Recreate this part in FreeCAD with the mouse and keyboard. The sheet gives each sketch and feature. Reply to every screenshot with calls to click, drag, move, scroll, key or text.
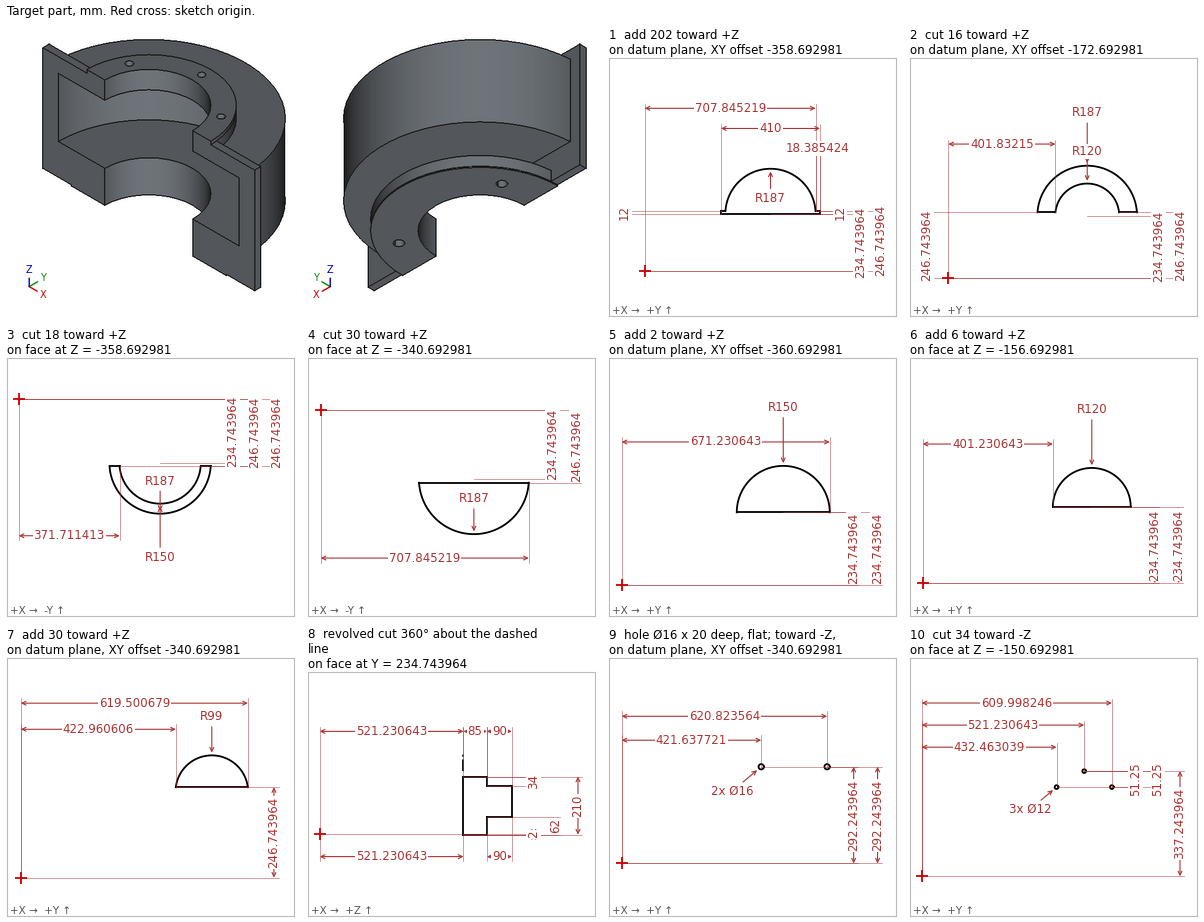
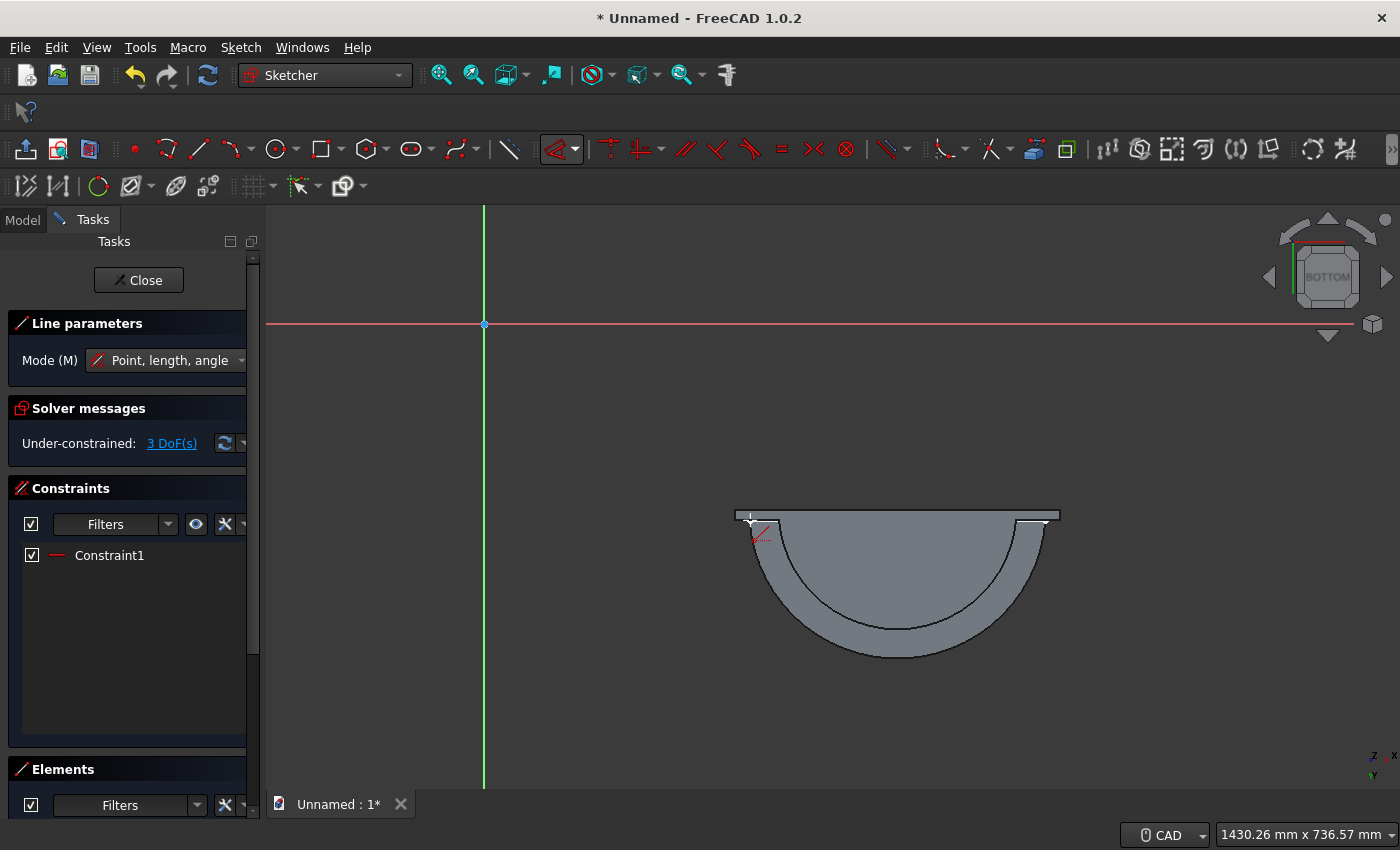
key(g)
key(3)
key(a)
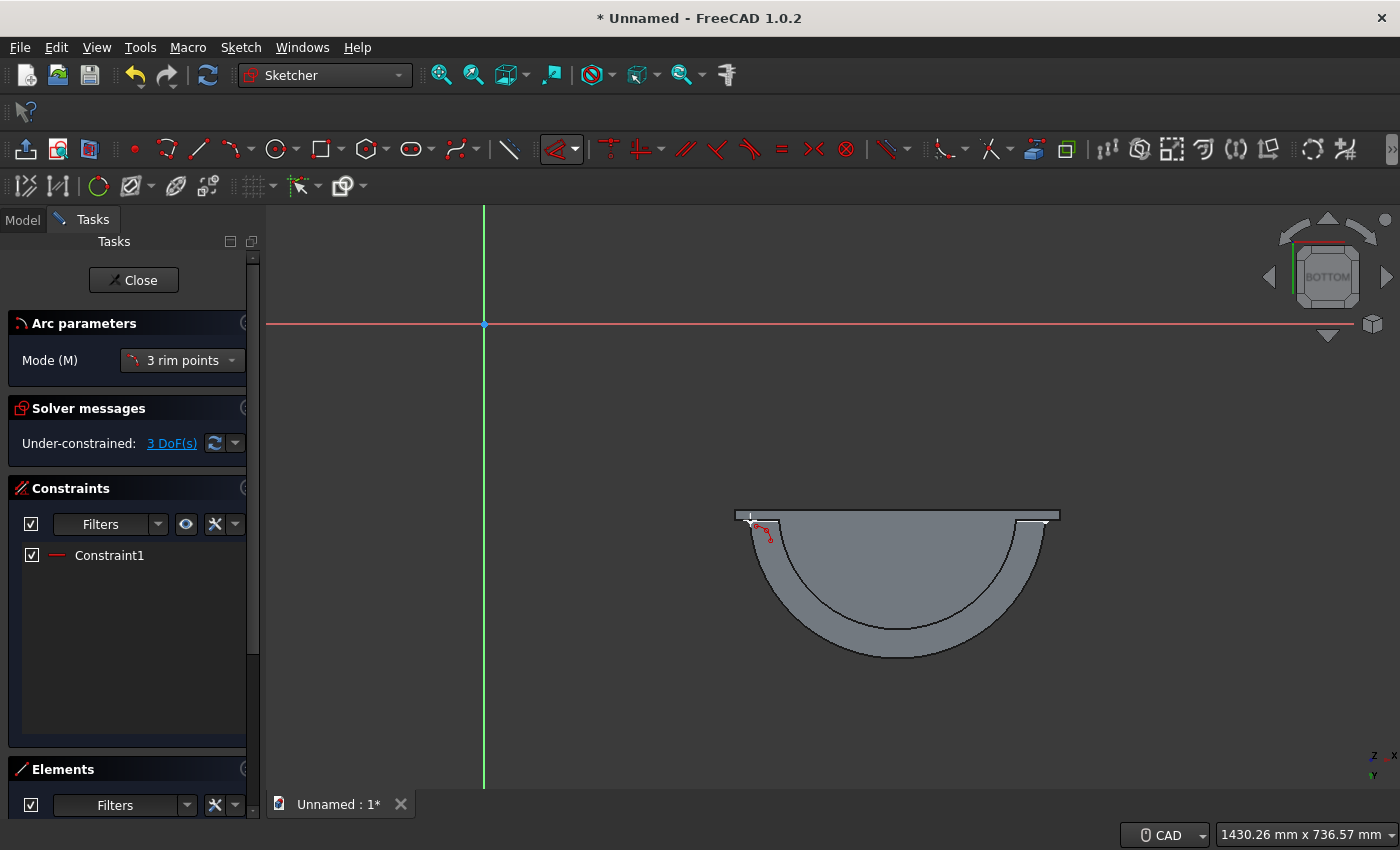
click(750, 521)
click(1045, 521)
click(898, 659)
key(Escape)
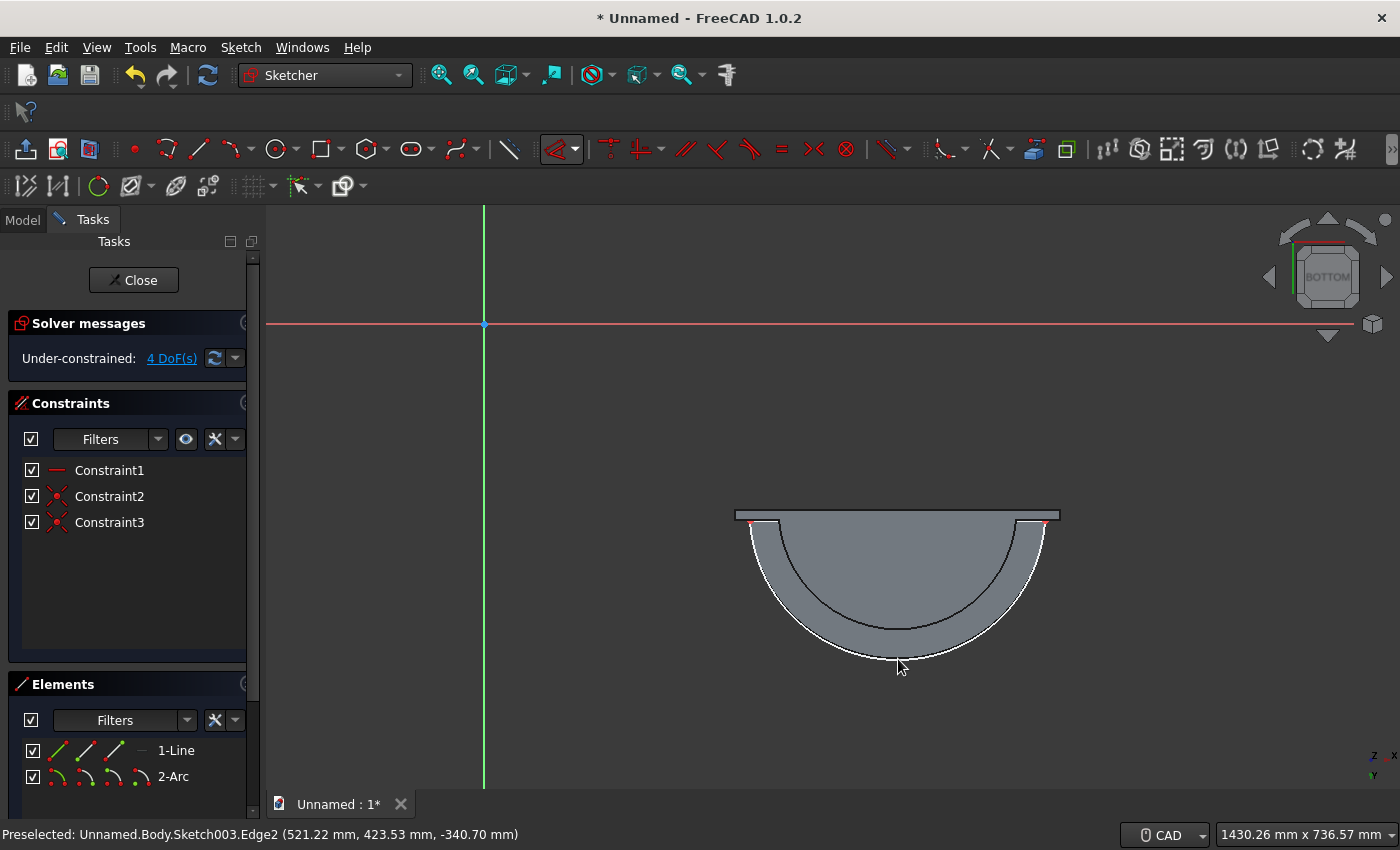
key(d)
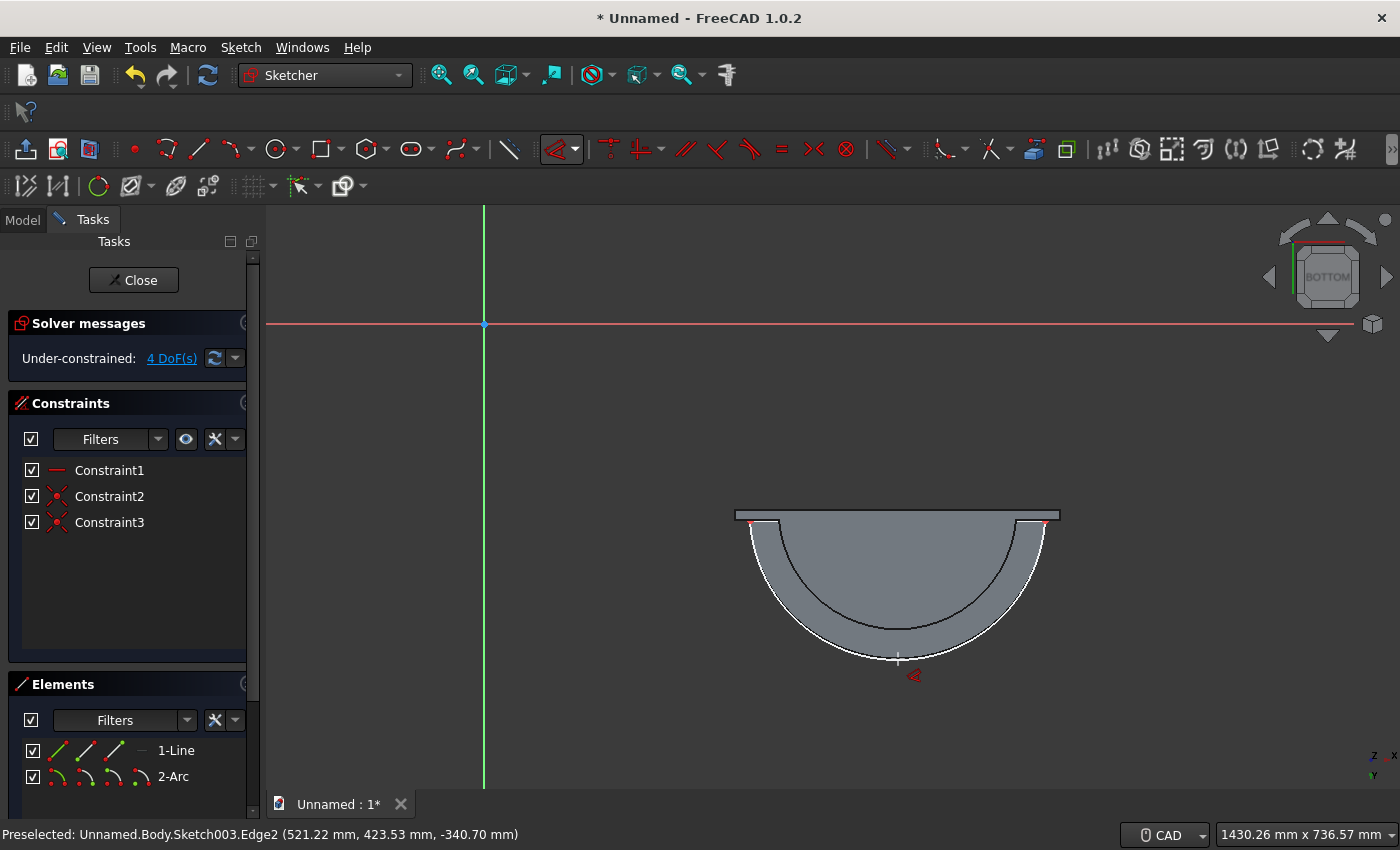
click(814, 634)
click(796, 660)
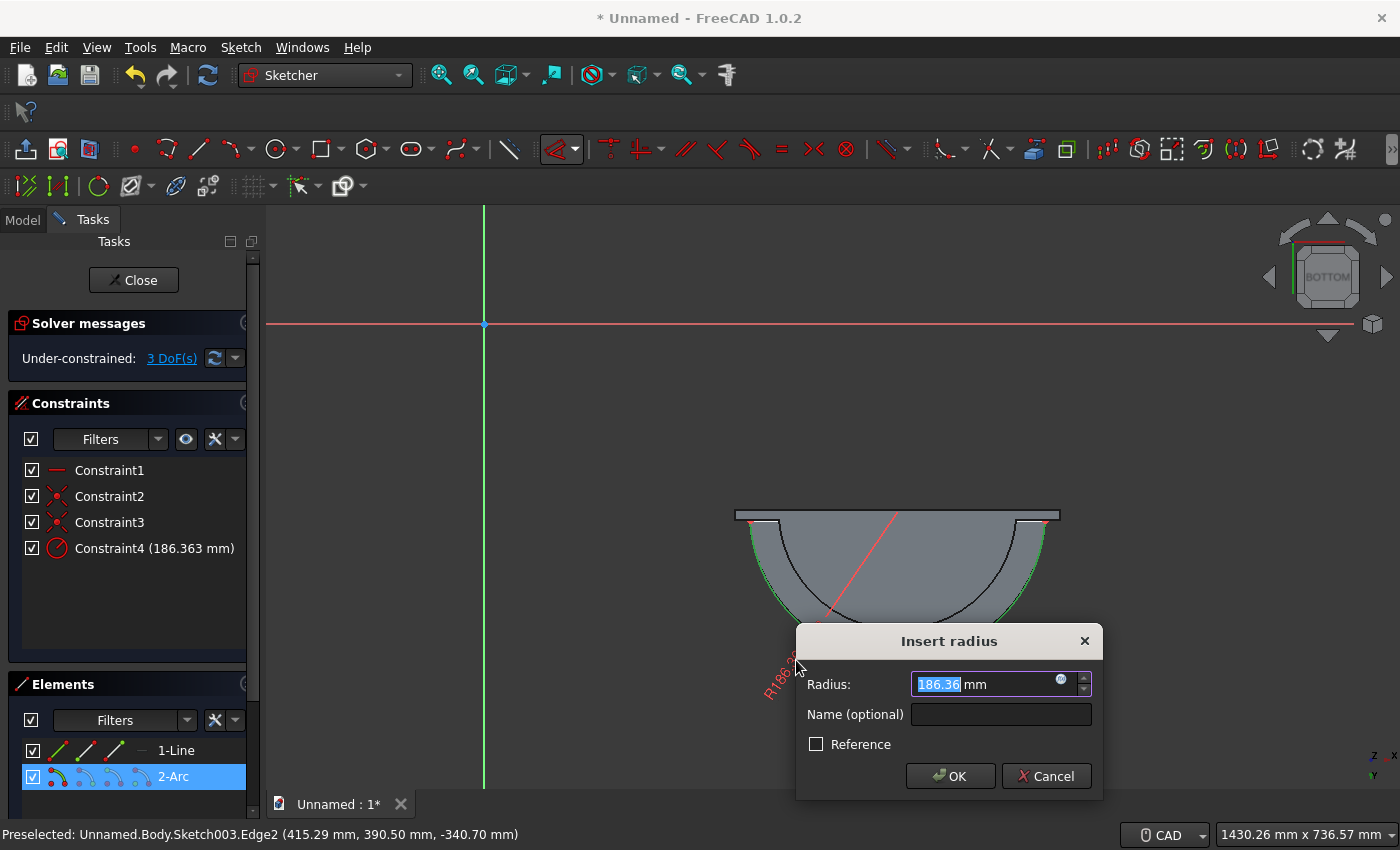
text(187)
key(Return)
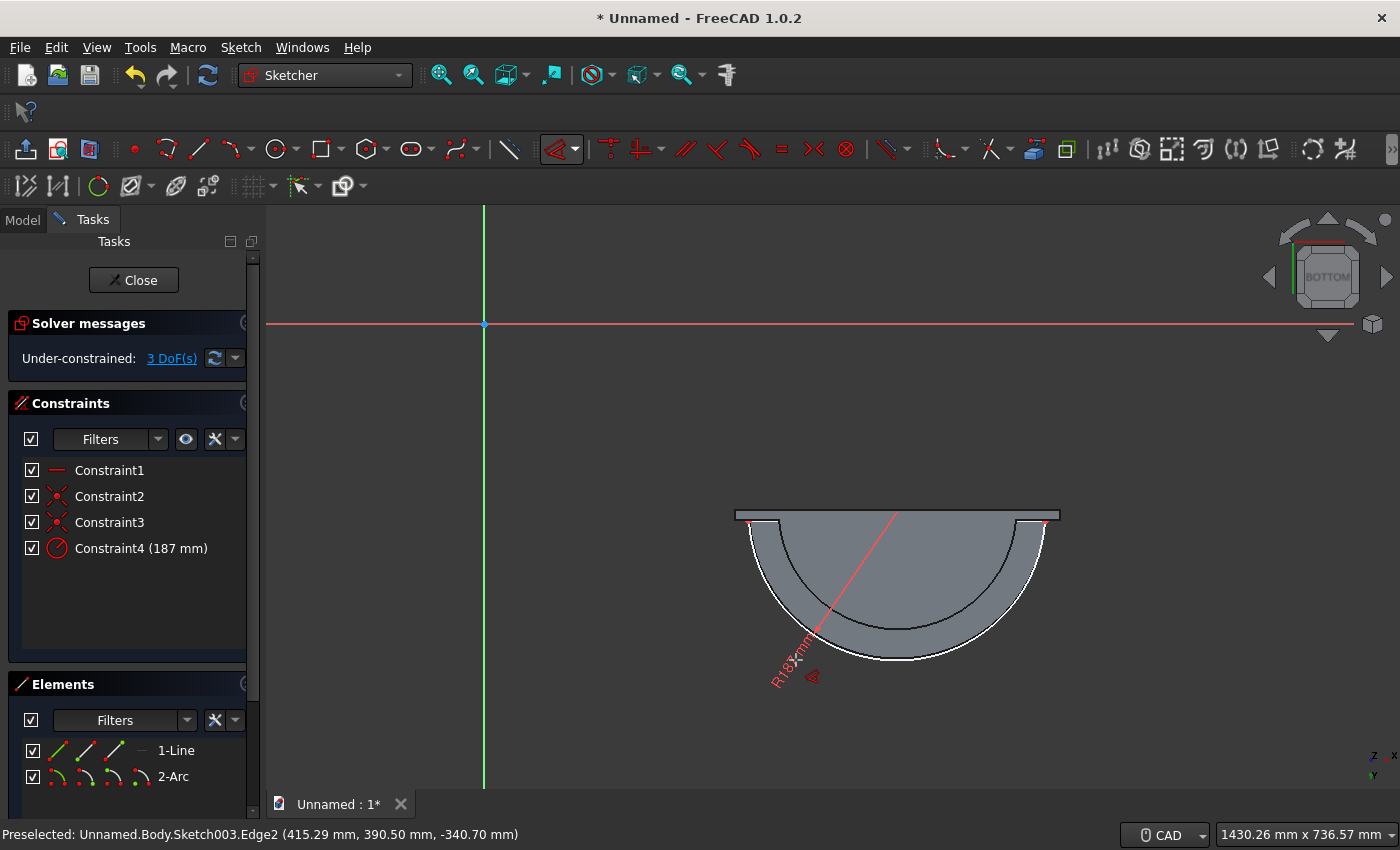
click(1045, 521)
click(765, 290)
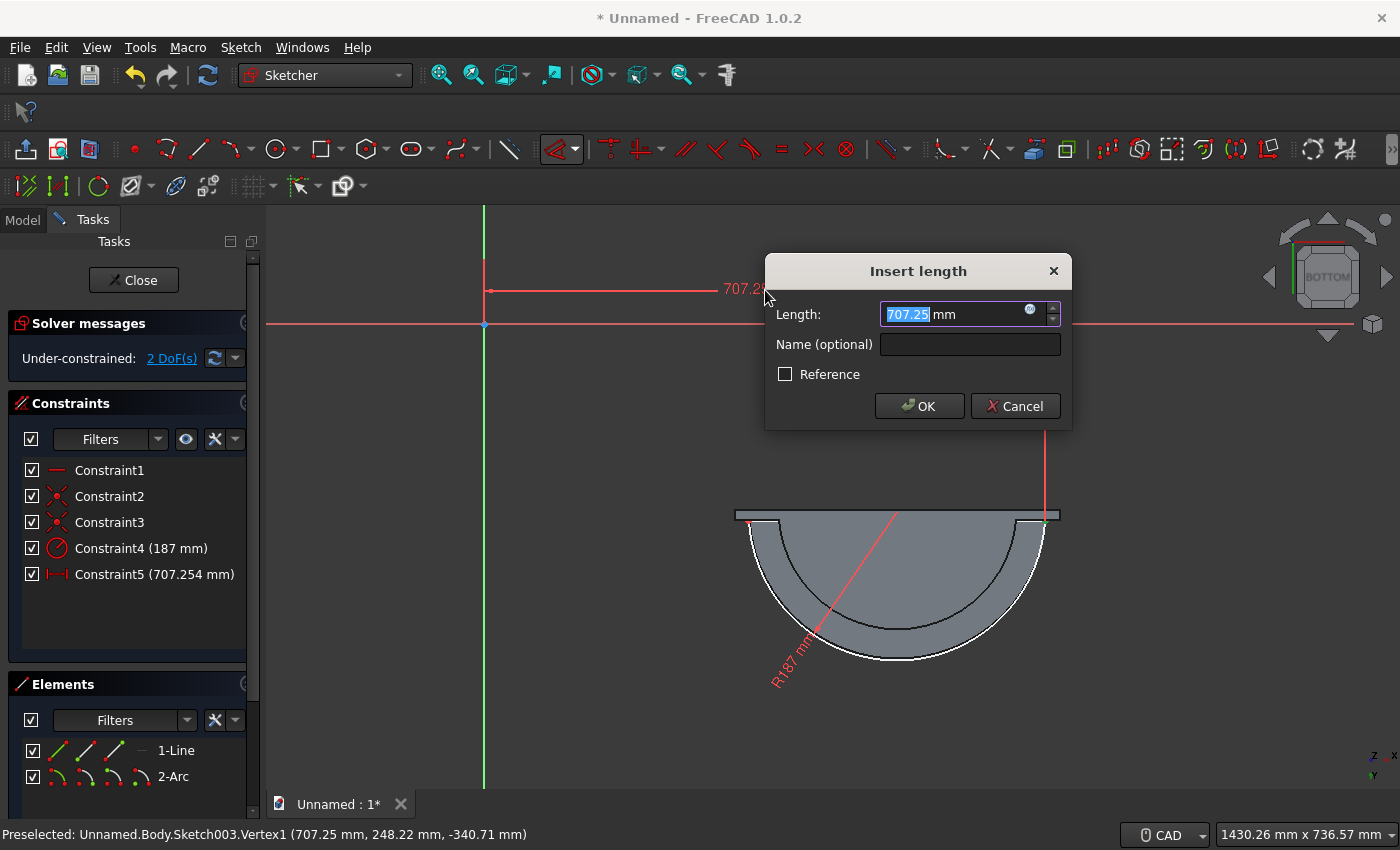
text(707.845219)
key(Return)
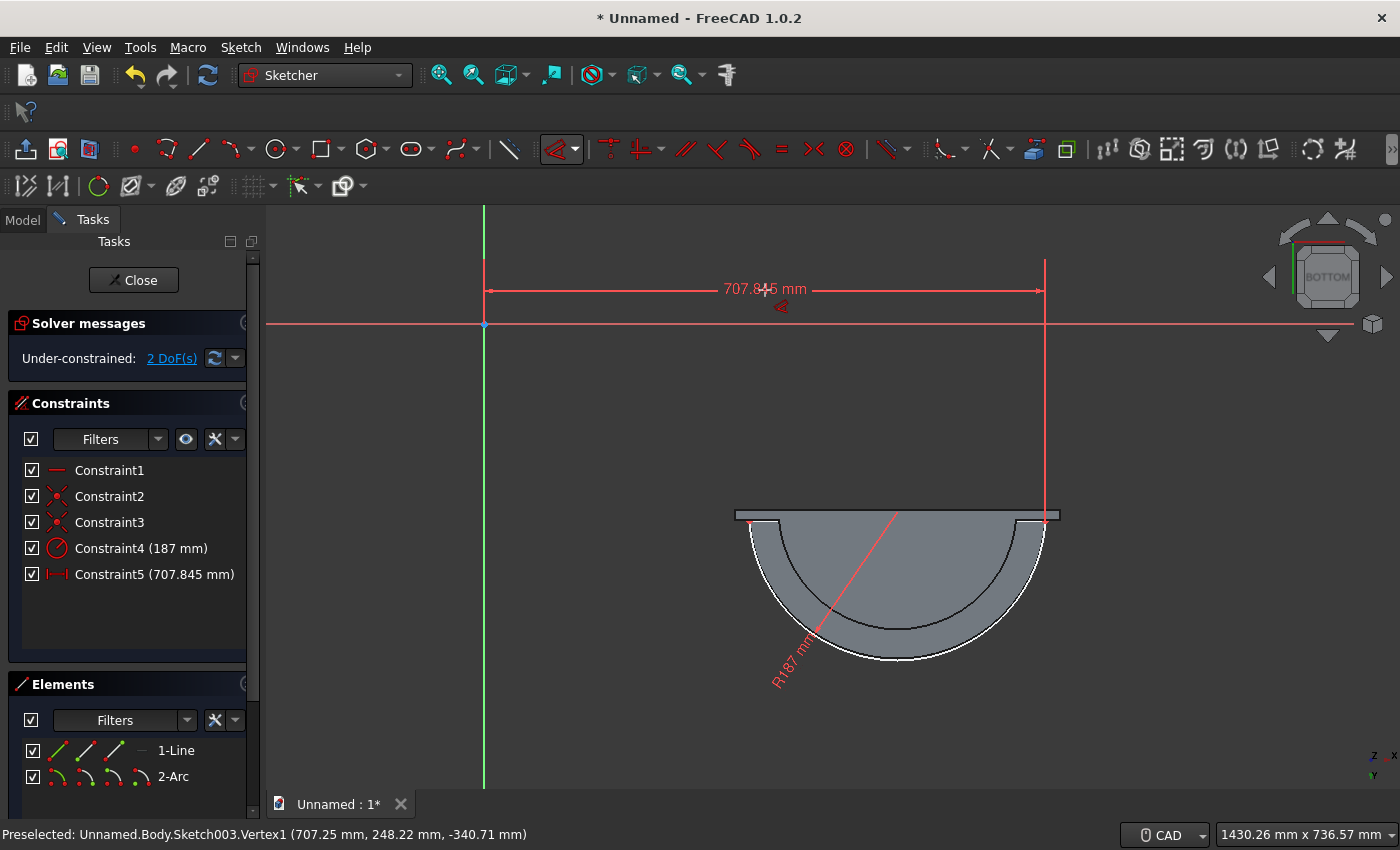
click(1045, 521)
click(1079, 423)